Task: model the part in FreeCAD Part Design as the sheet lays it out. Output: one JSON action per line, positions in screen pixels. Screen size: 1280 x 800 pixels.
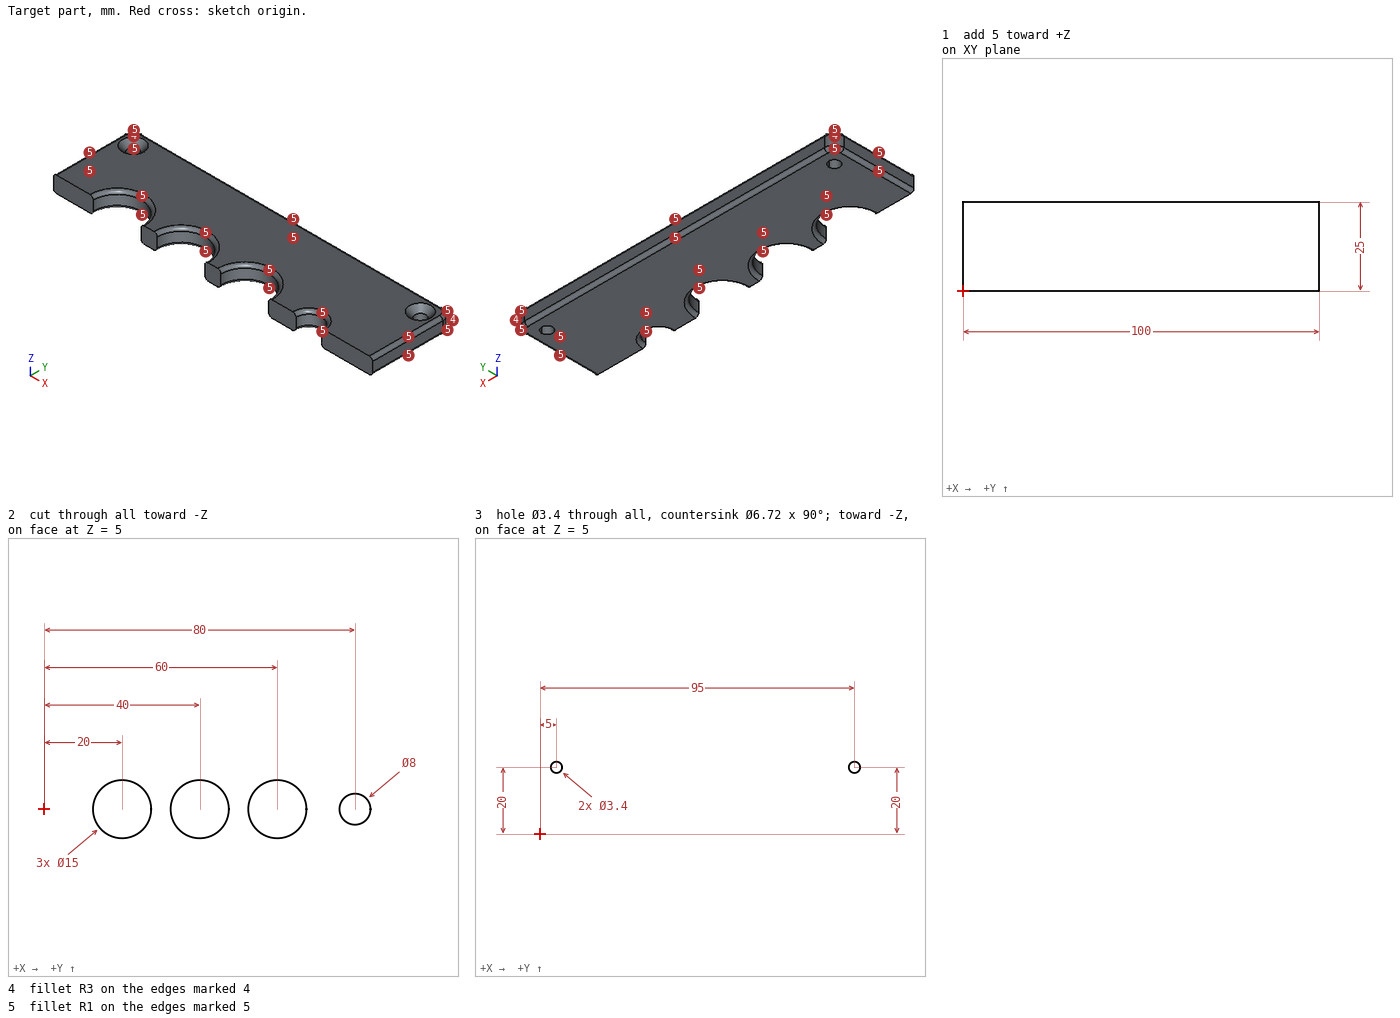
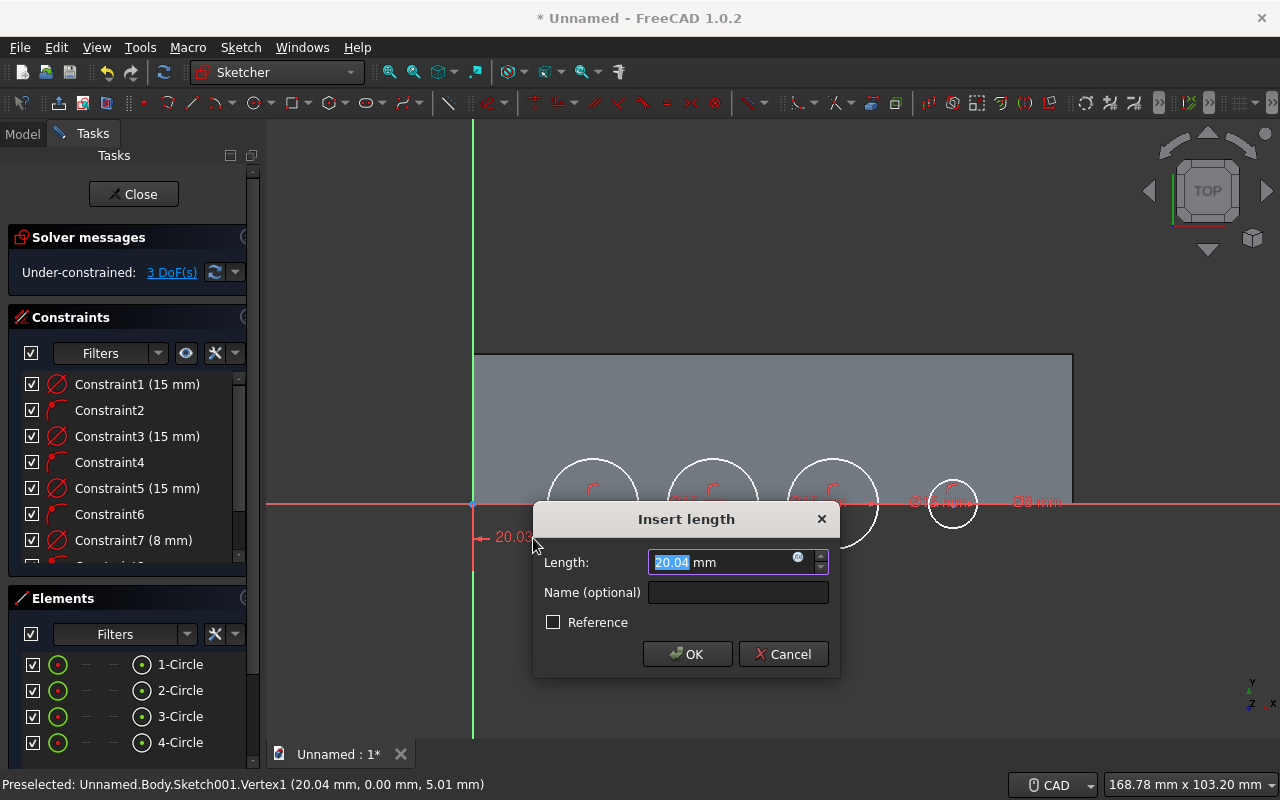
{"action": "type", "text": "20"}
{"action": "key", "text": "Return"}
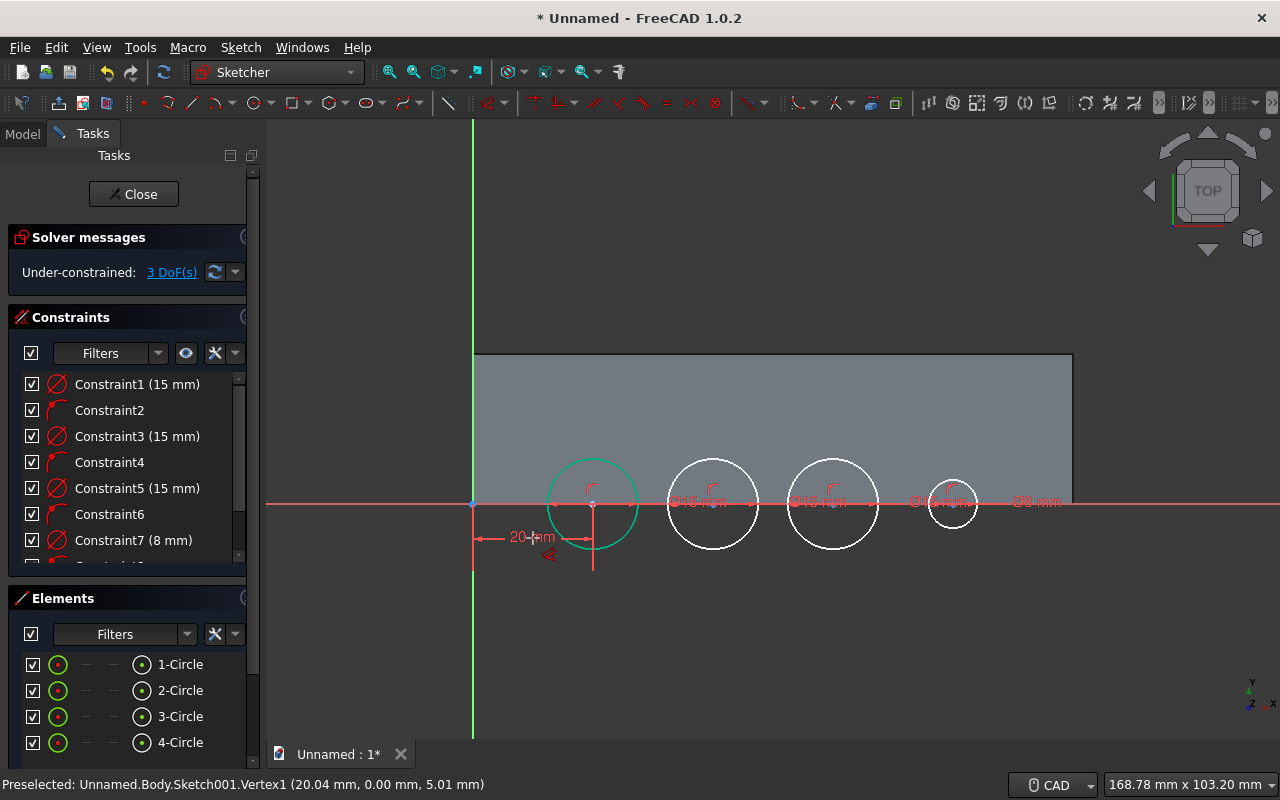
{"action": "left_click", "coordinate": [713, 504]}
{"action": "left_click", "coordinate": [648, 538]}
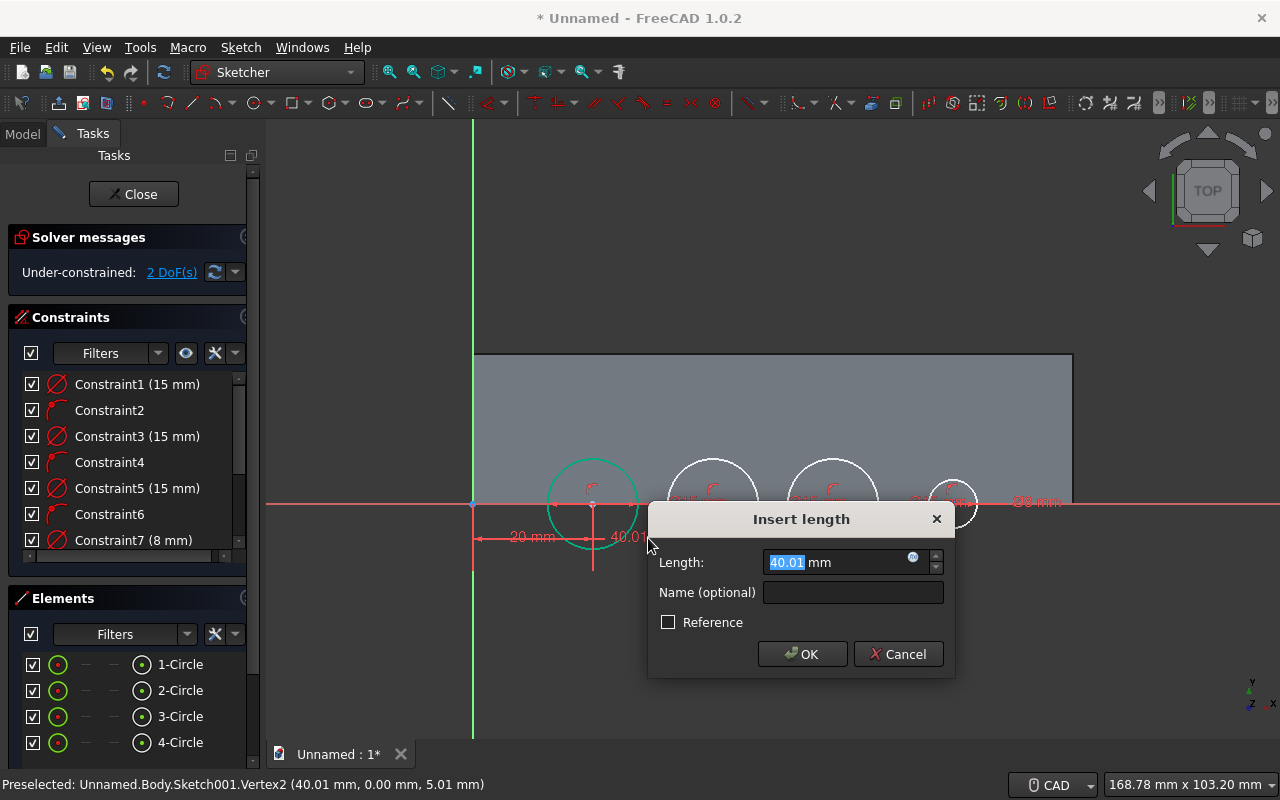
{"action": "type", "text": "40"}
{"action": "key", "text": "Return"}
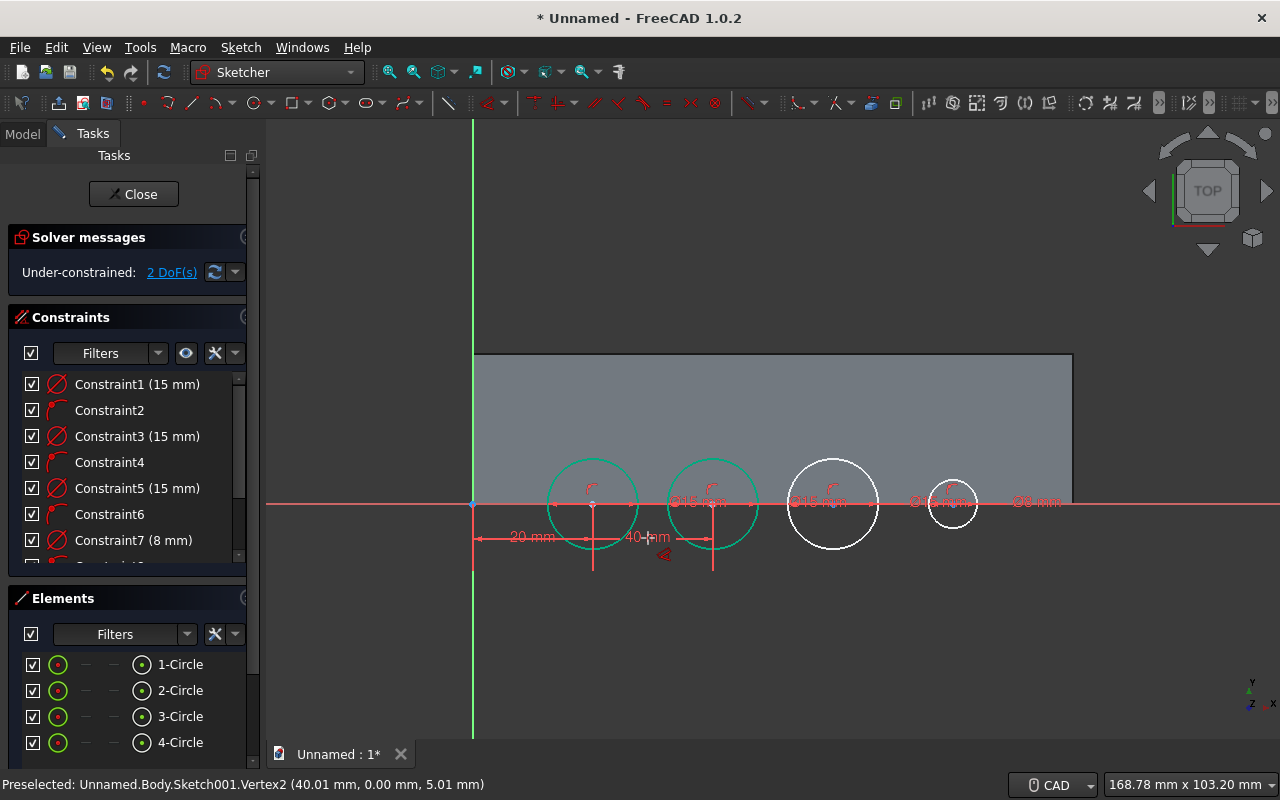
{"action": "left_click", "coordinate": [833, 504]}
{"action": "left_click", "coordinate": [779, 538]}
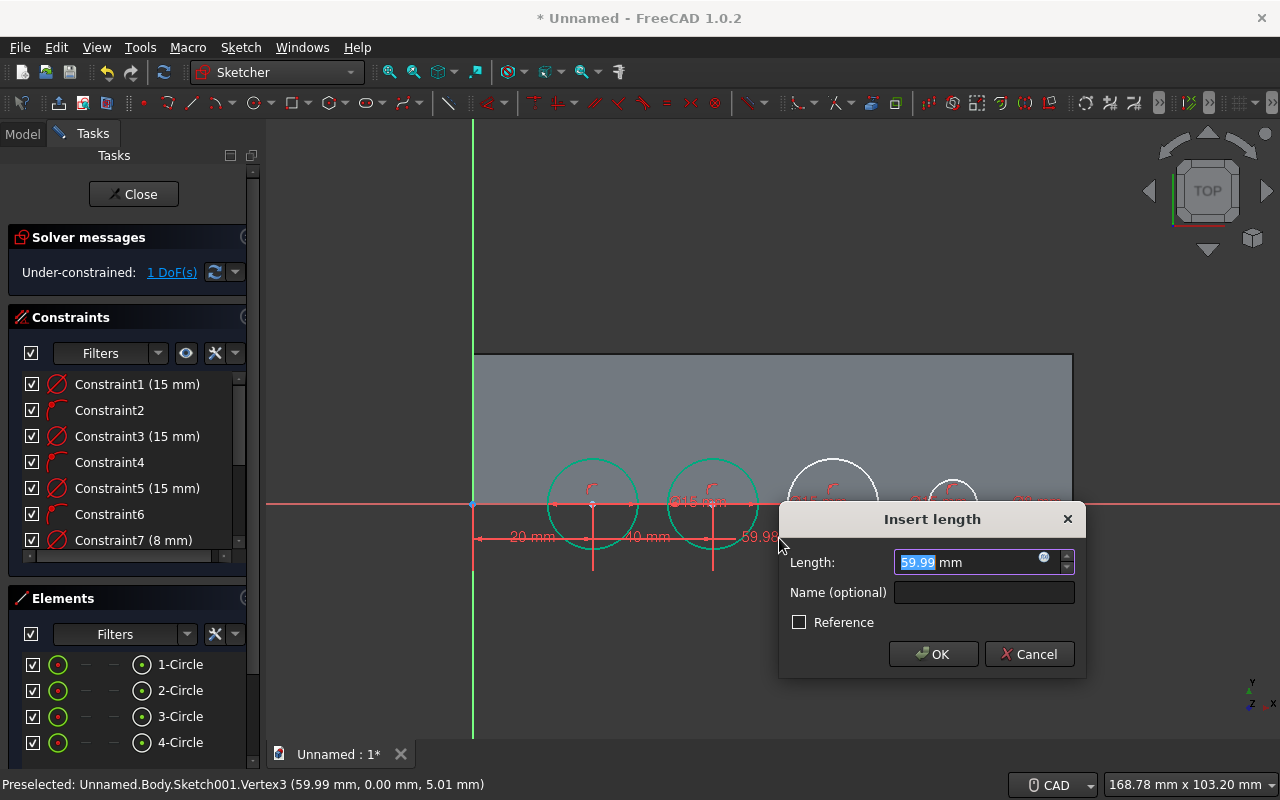
{"action": "type", "text": "60"}
{"action": "key", "text": "Return"}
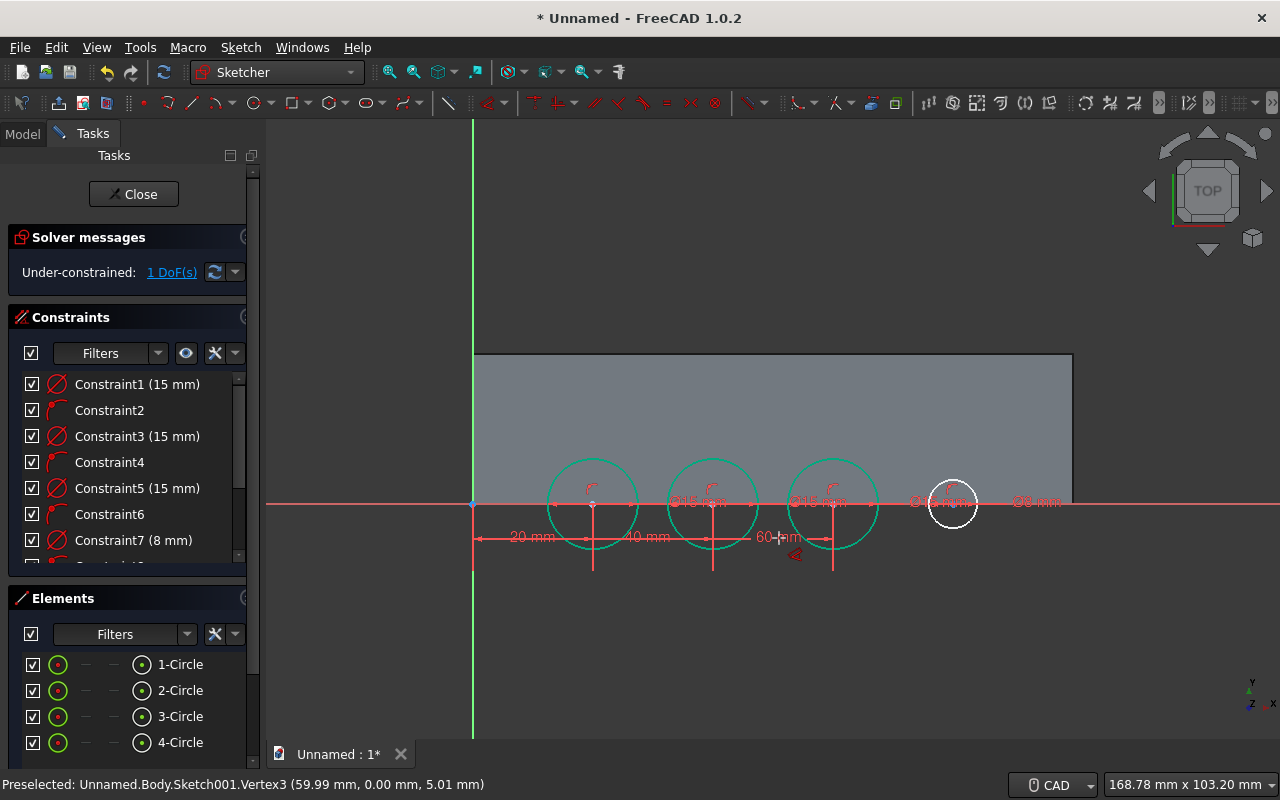
{"action": "left_click", "coordinate": [953, 504]}
{"action": "left_click", "coordinate": [881, 538]}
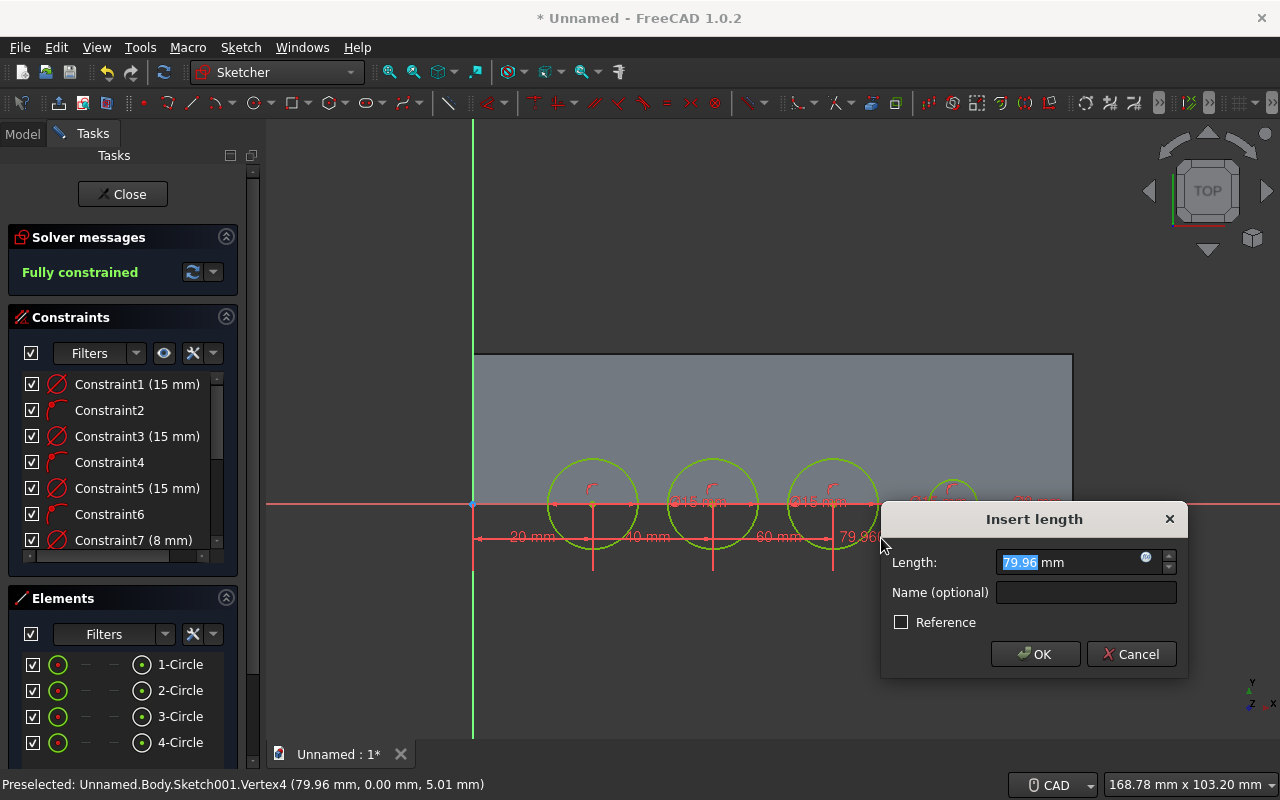
{"action": "type", "text": "80"}
{"action": "key", "text": "Return"}
{"action": "key", "text": "Escape"}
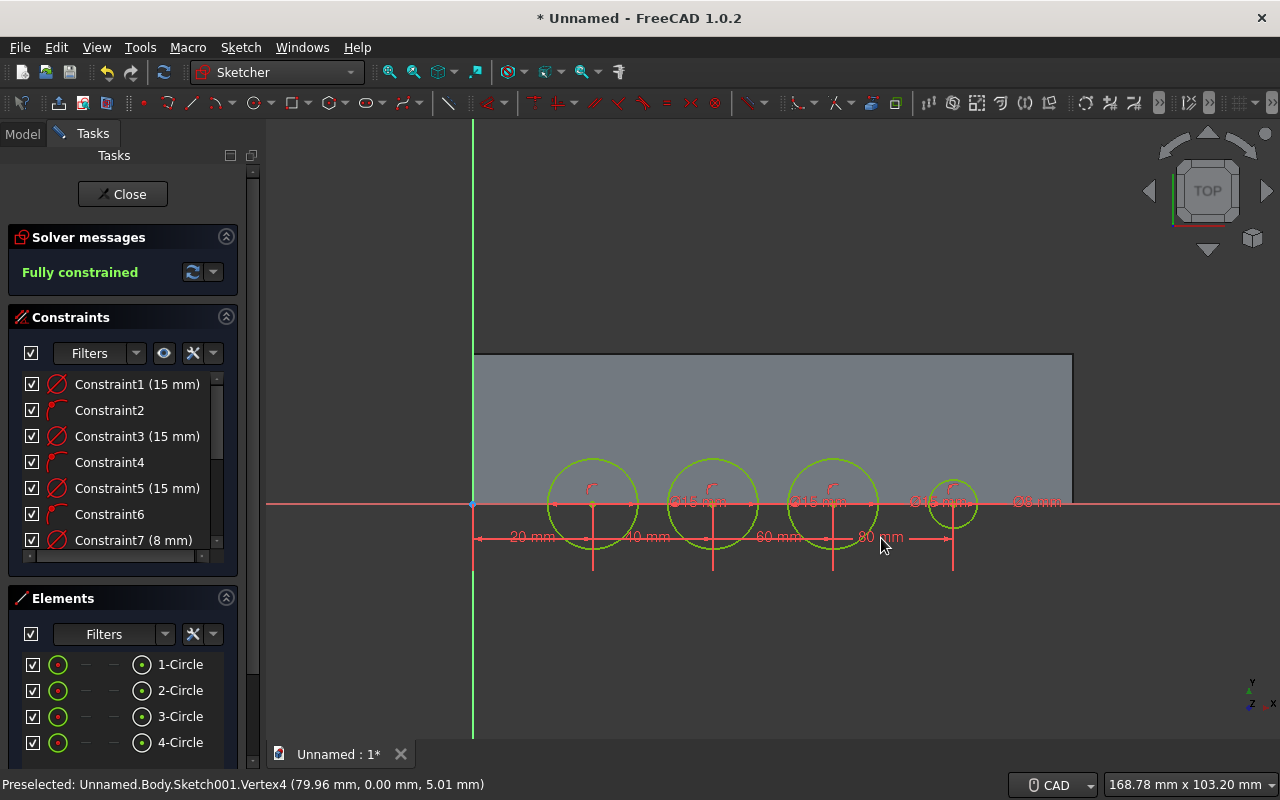
{"action": "left_click", "coordinate": [123, 194]}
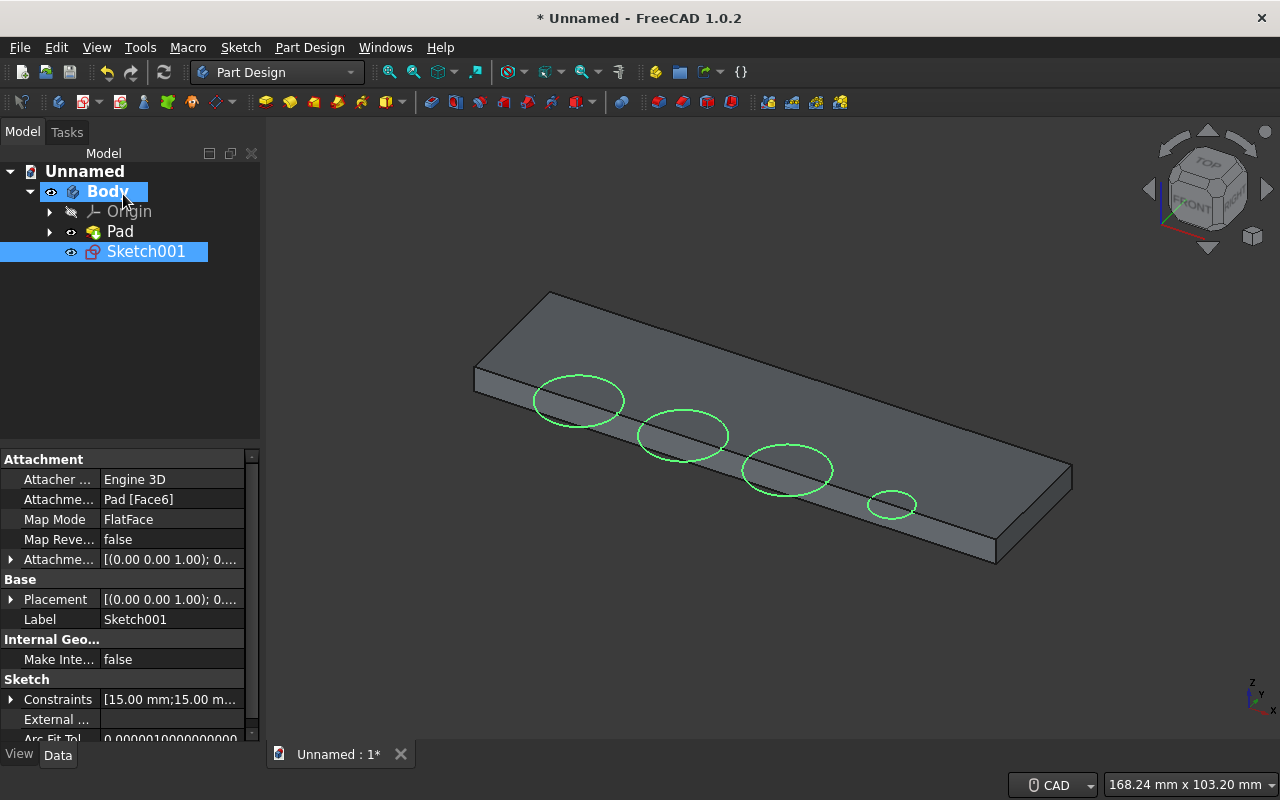
{"action": "left_click", "coordinate": [432, 102]}